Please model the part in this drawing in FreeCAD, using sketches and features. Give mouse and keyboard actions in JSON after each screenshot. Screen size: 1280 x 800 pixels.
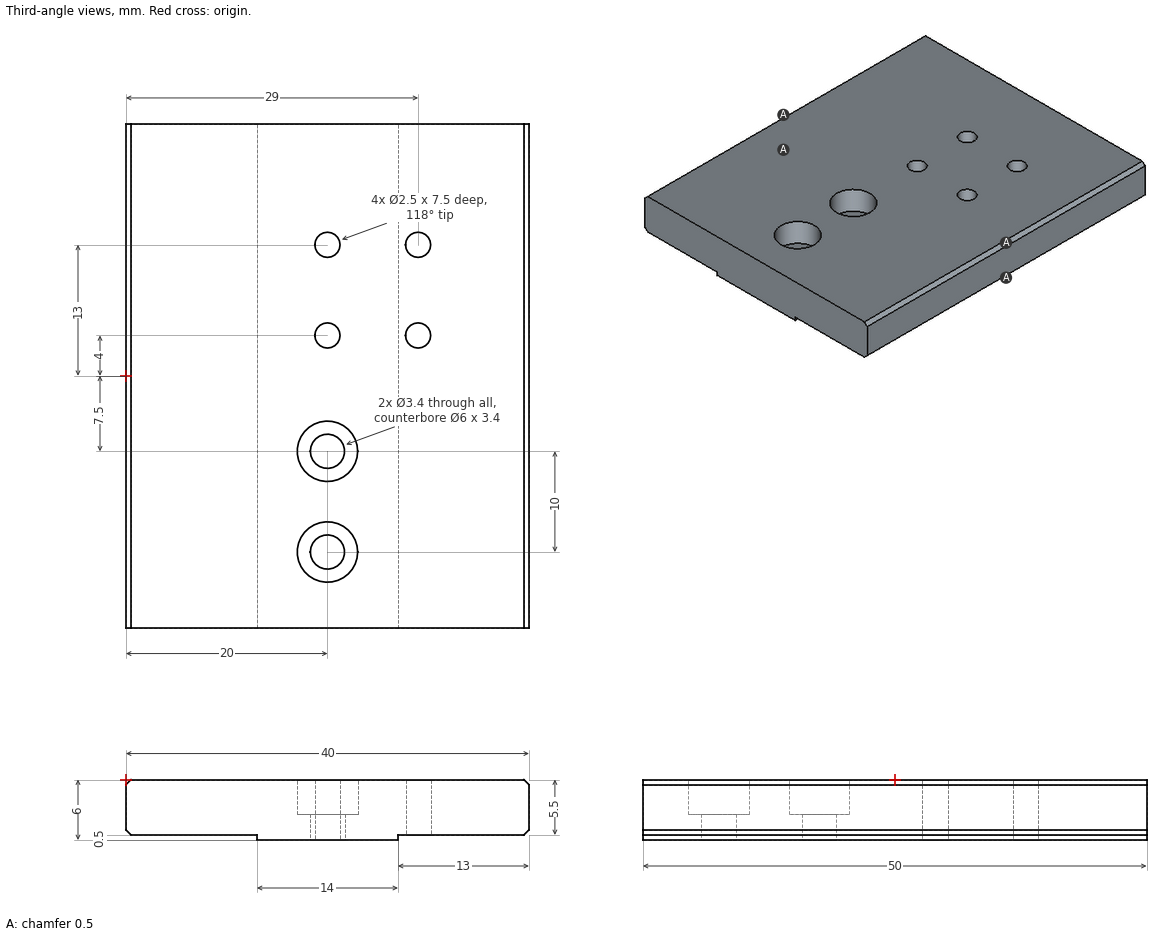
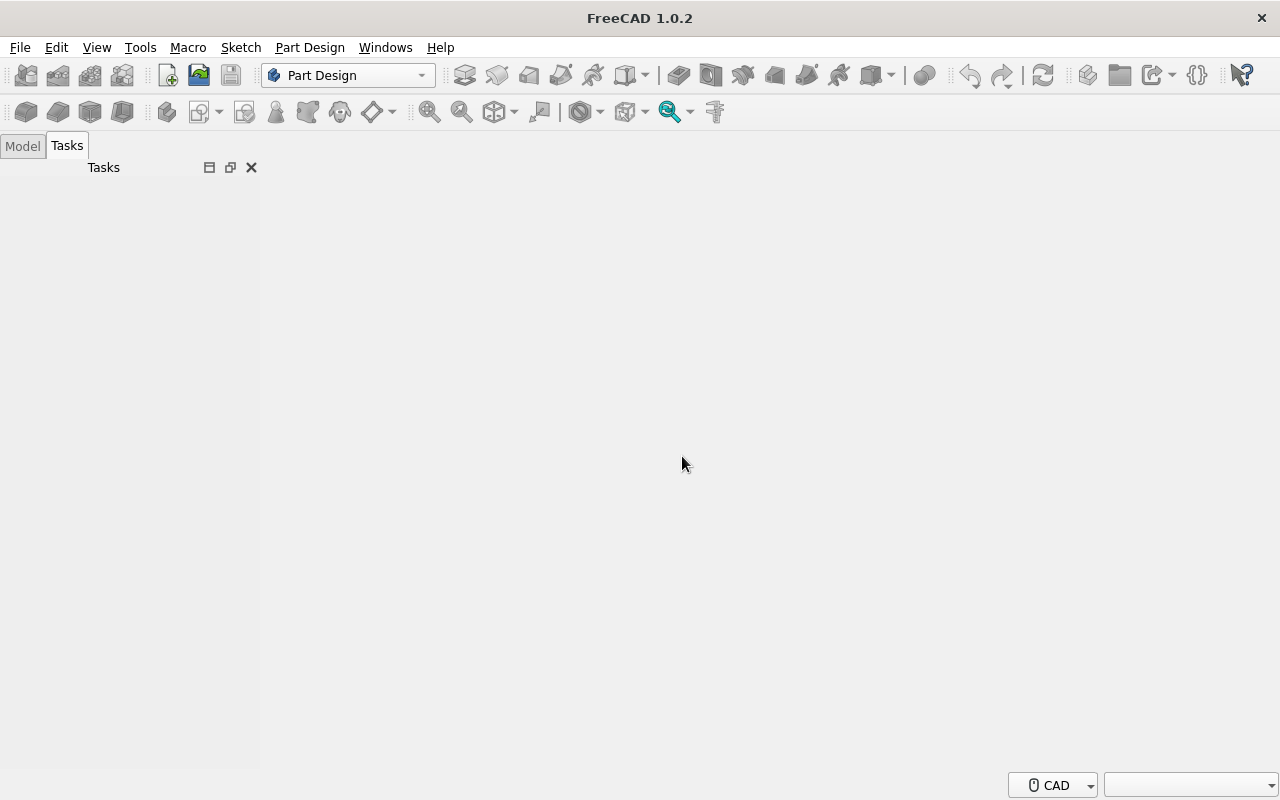
{"action": "left_click", "coordinate": [168, 76]}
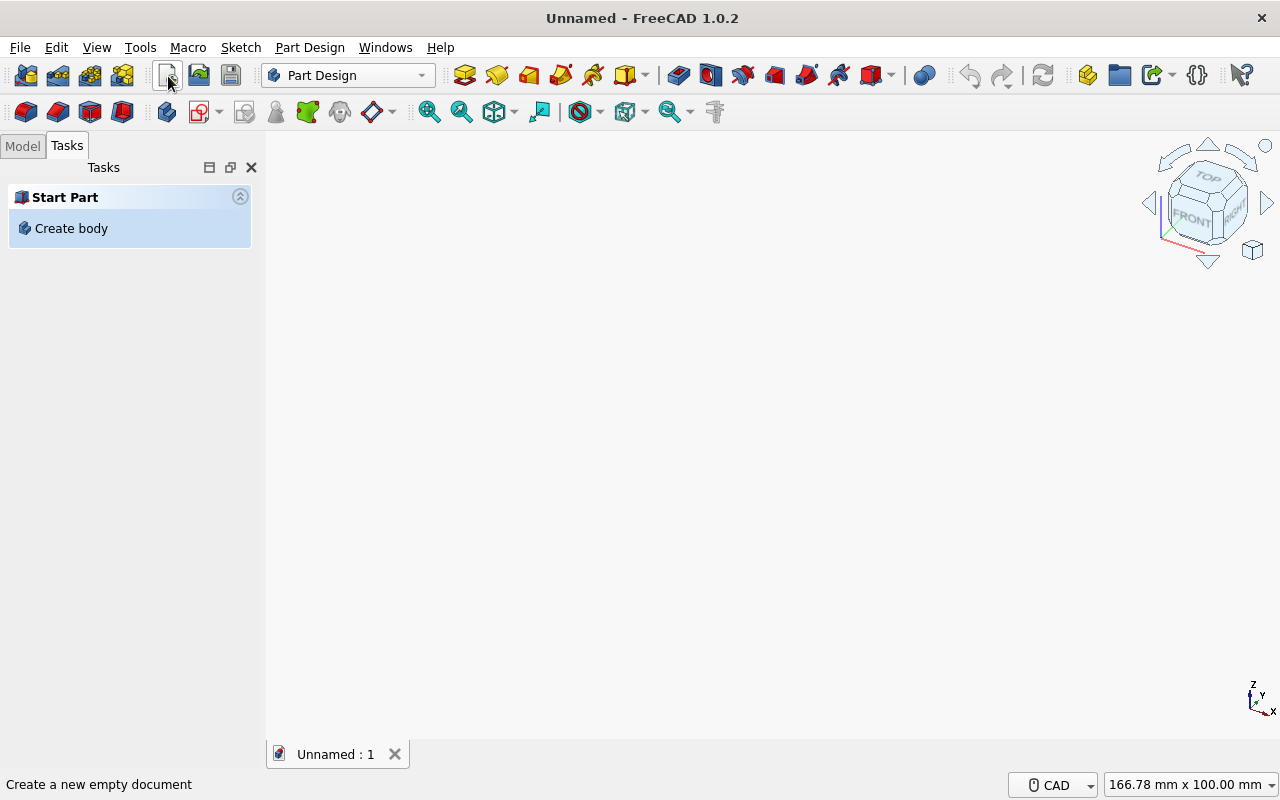
{"action": "left_click", "coordinate": [200, 112]}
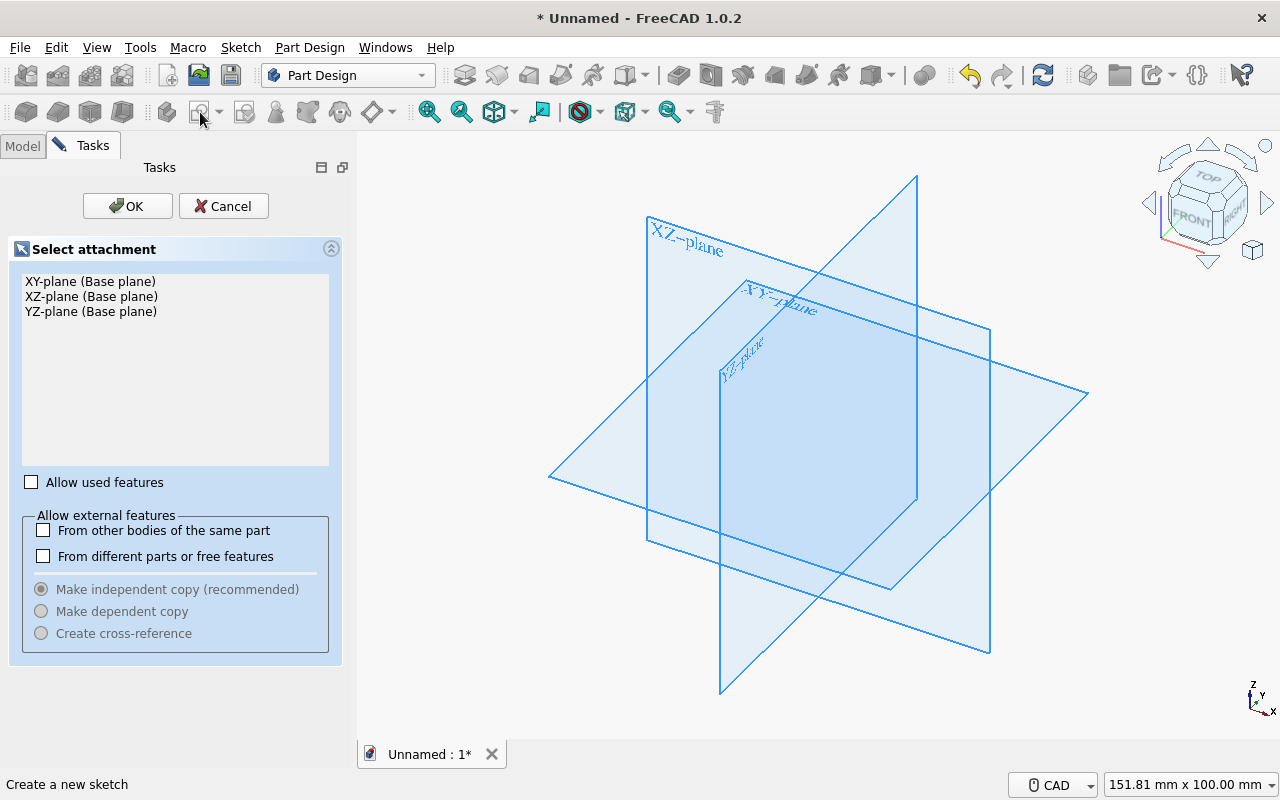
{"action": "left_click", "coordinate": [82, 296]}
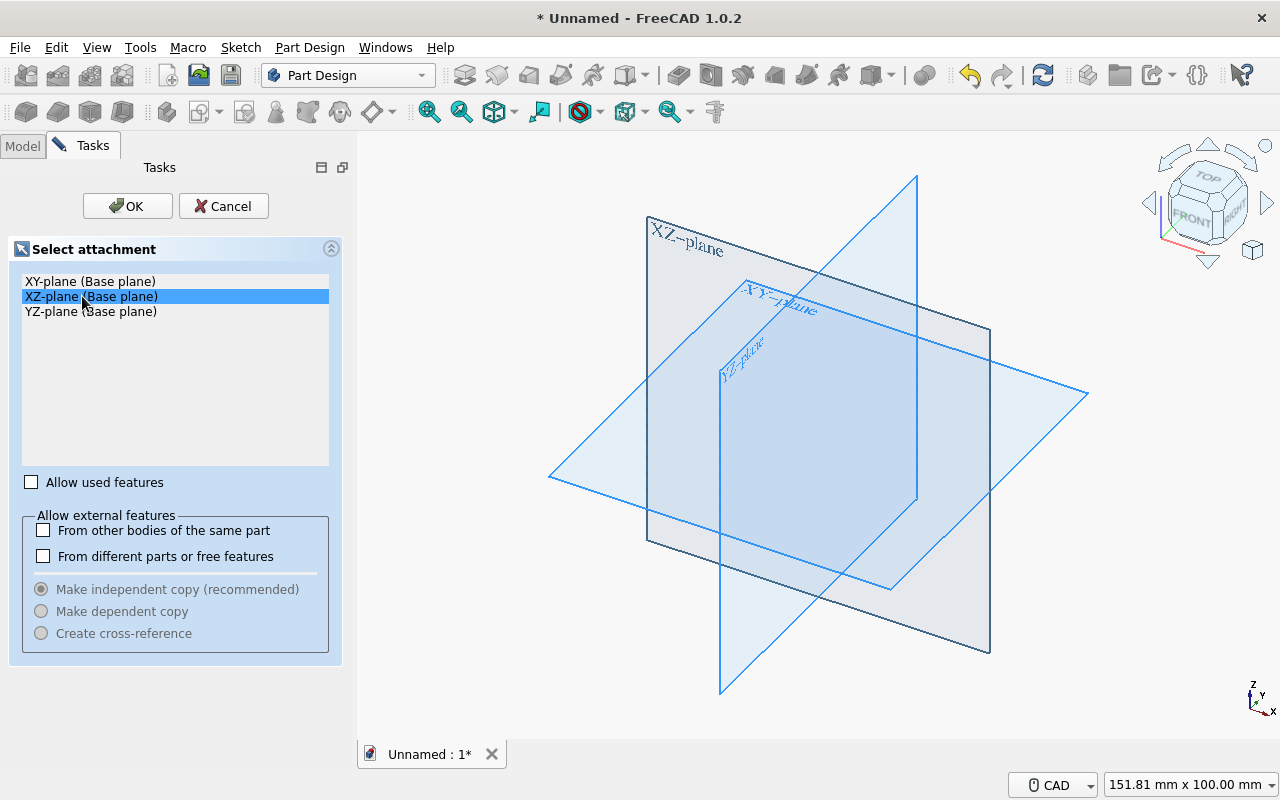
{"action": "left_click", "coordinate": [128, 206]}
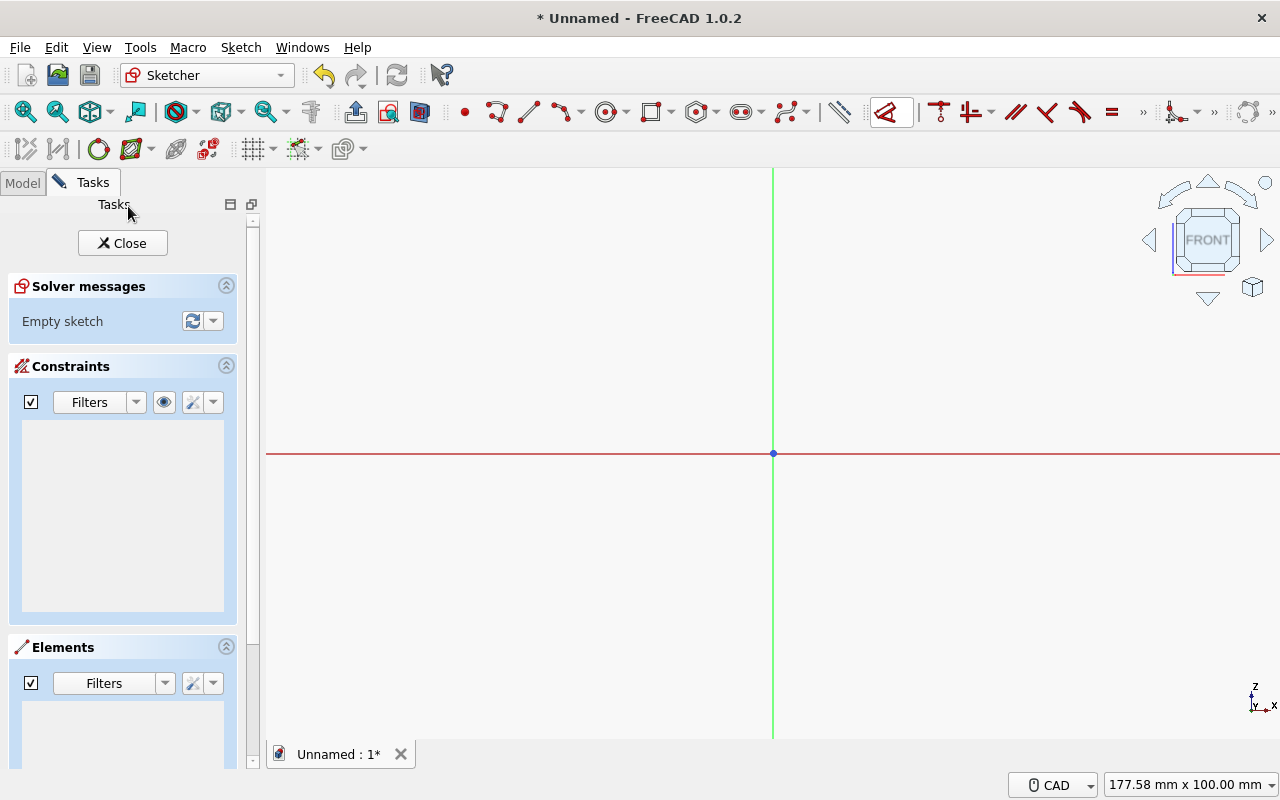
{"action": "scroll", "coordinate": [994, 481], "scroll_direction": "up", "scroll_amount": 5}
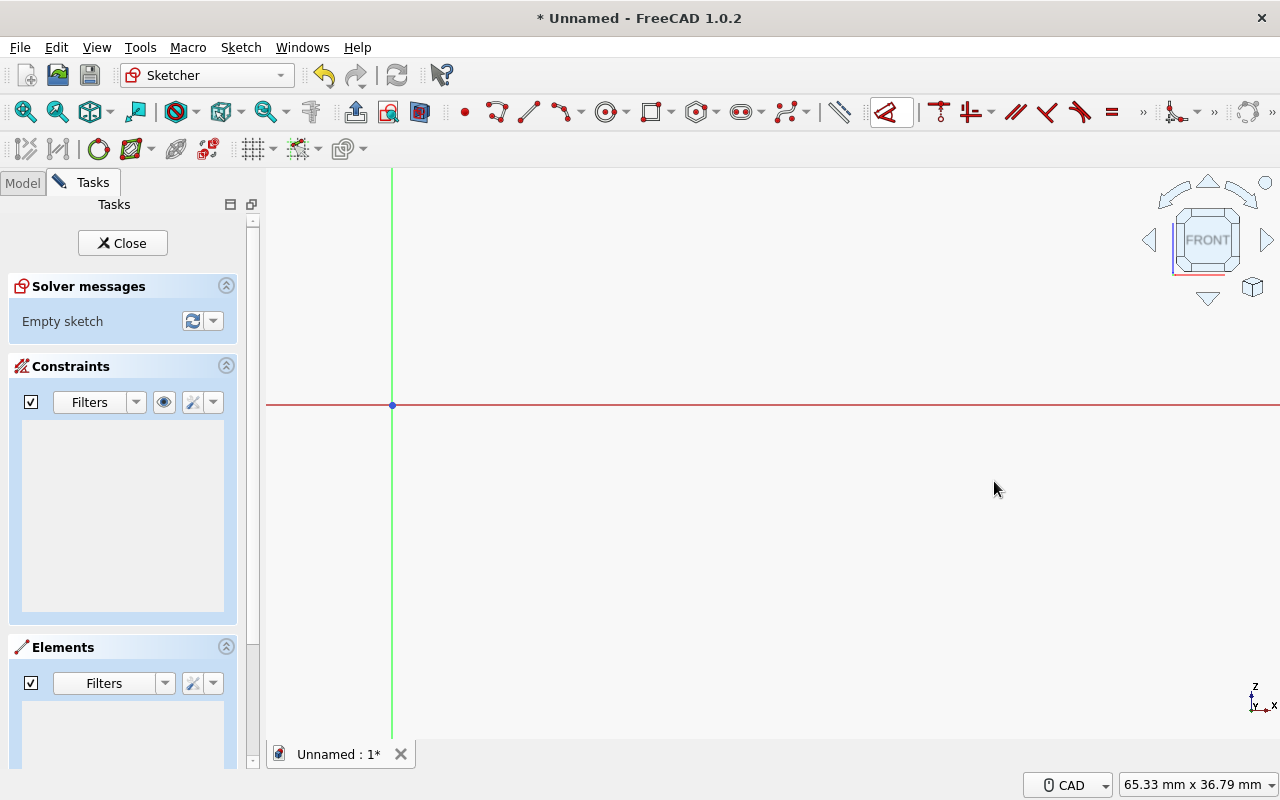
{"action": "key", "text": "g m"}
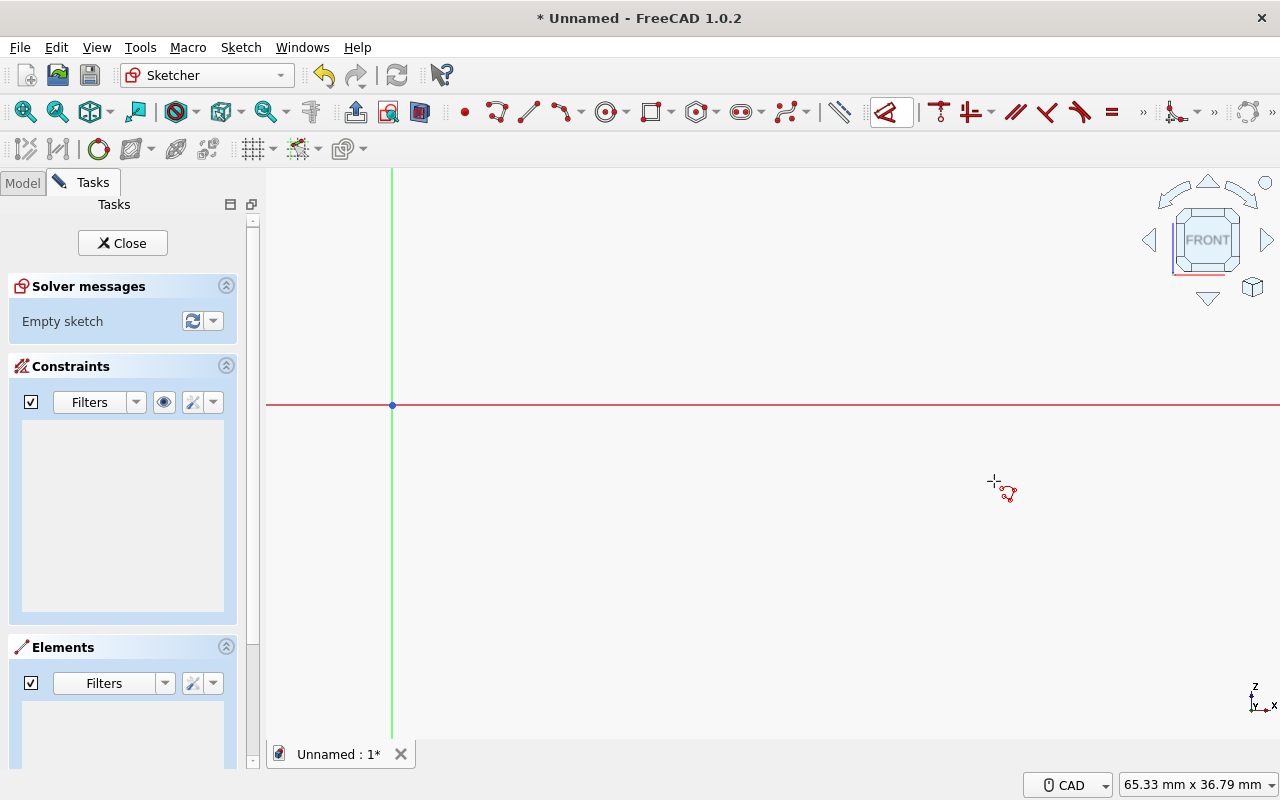
{"action": "left_click", "coordinate": [392, 405]}
{"action": "left_click", "coordinate": [1013, 414]}
{"action": "left_click", "coordinate": [1013, 491]}
{"action": "left_click", "coordinate": [811, 491]}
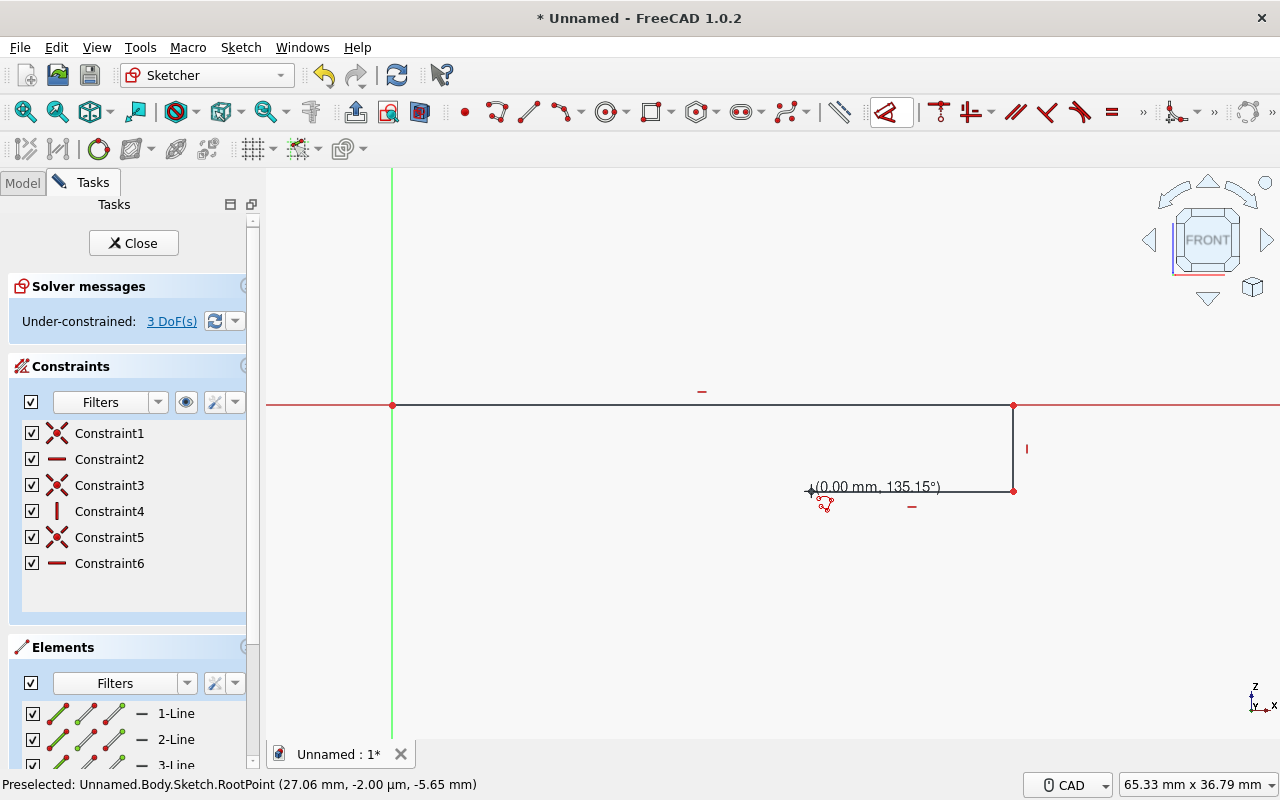
{"action": "scroll", "coordinate": [811, 498], "scroll_direction": "up", "scroll_amount": 4}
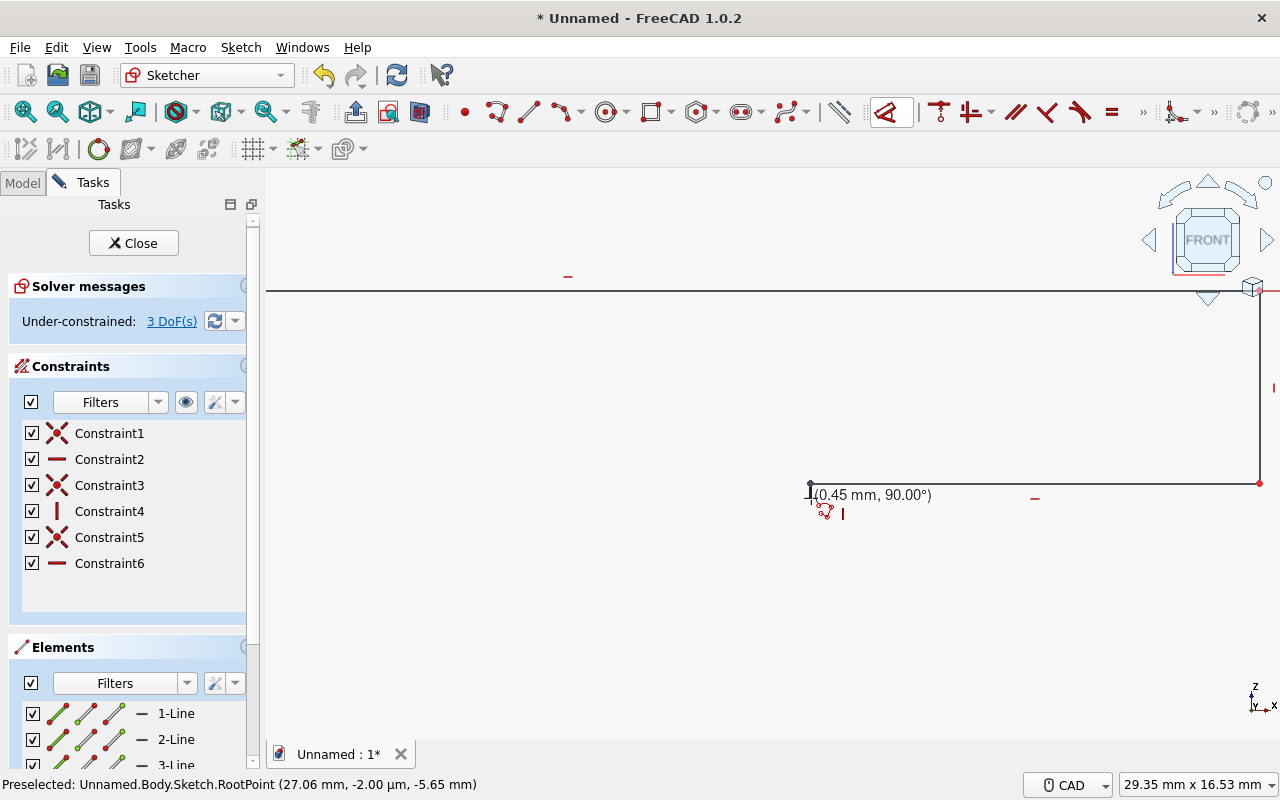
{"action": "left_click", "coordinate": [810, 498]}
{"action": "left_click", "coordinate": [327, 498]}
{"action": "left_click", "coordinate": [327, 481]}